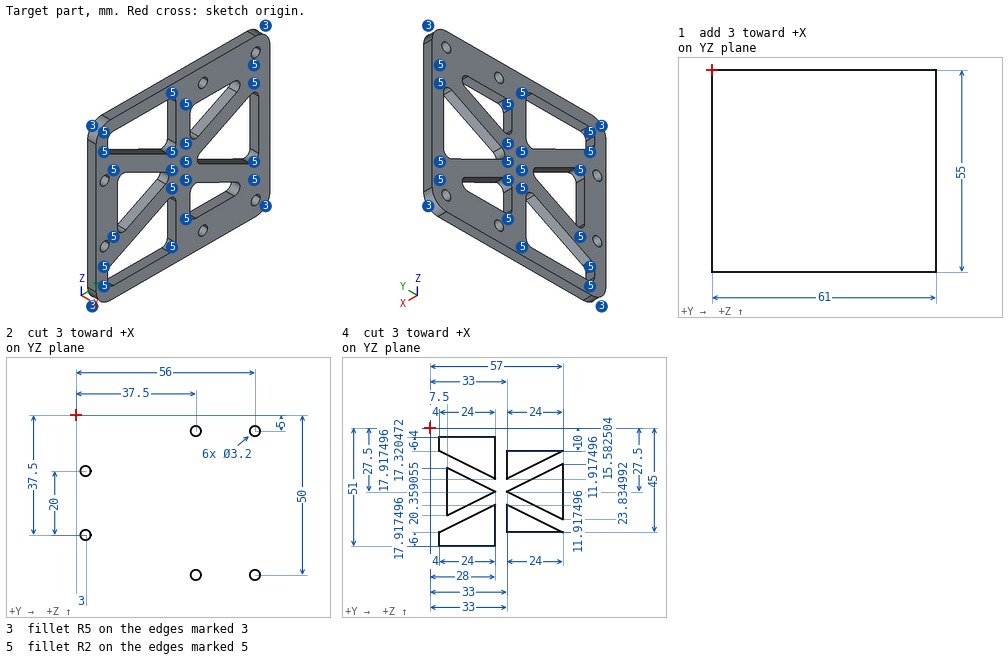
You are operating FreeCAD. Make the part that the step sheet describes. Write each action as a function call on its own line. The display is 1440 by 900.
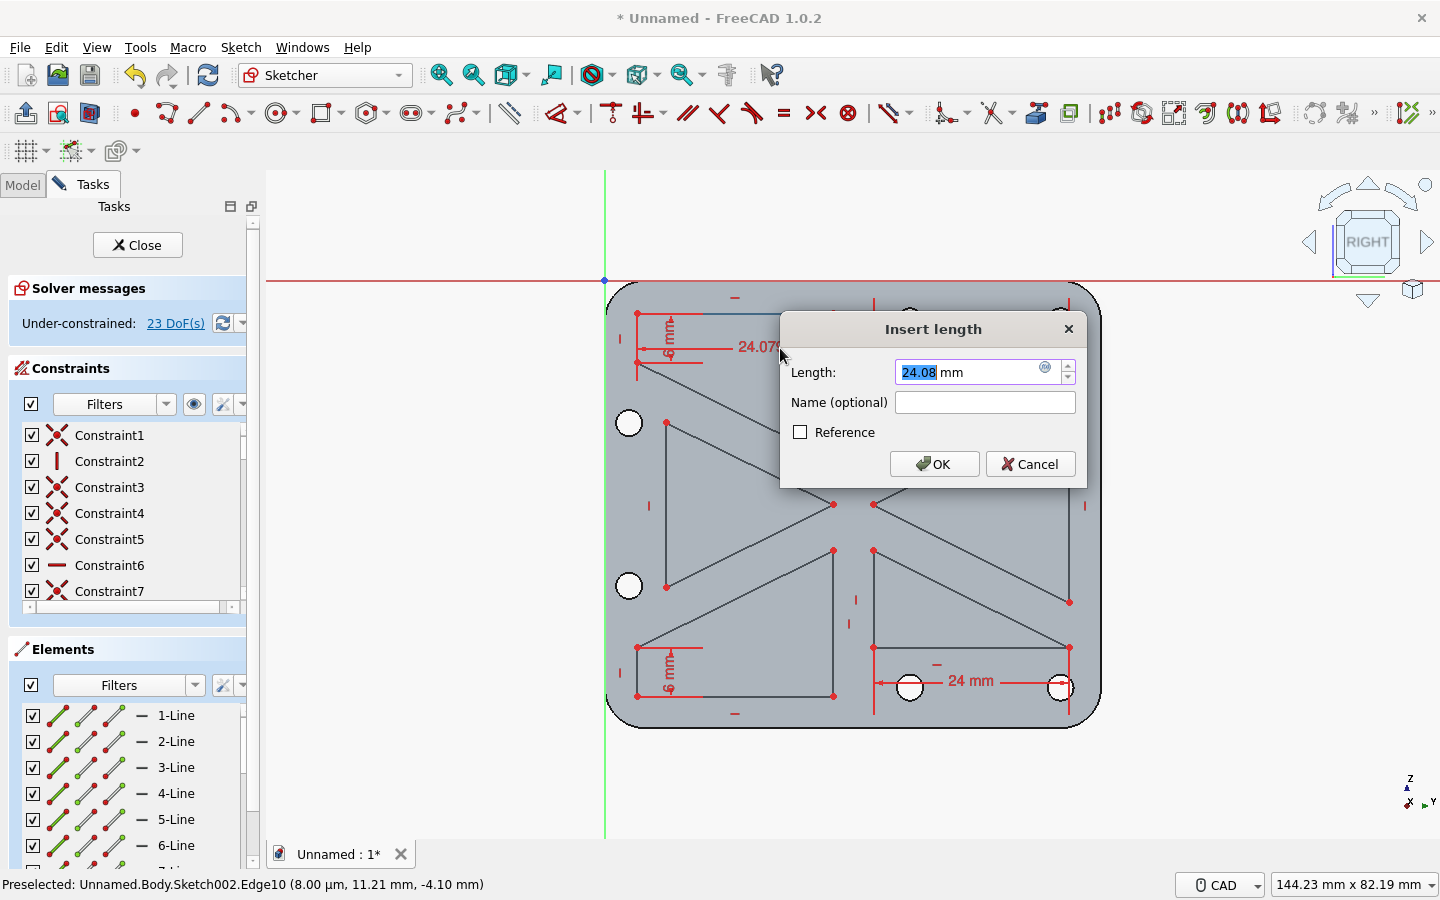
text(24)
key(Return)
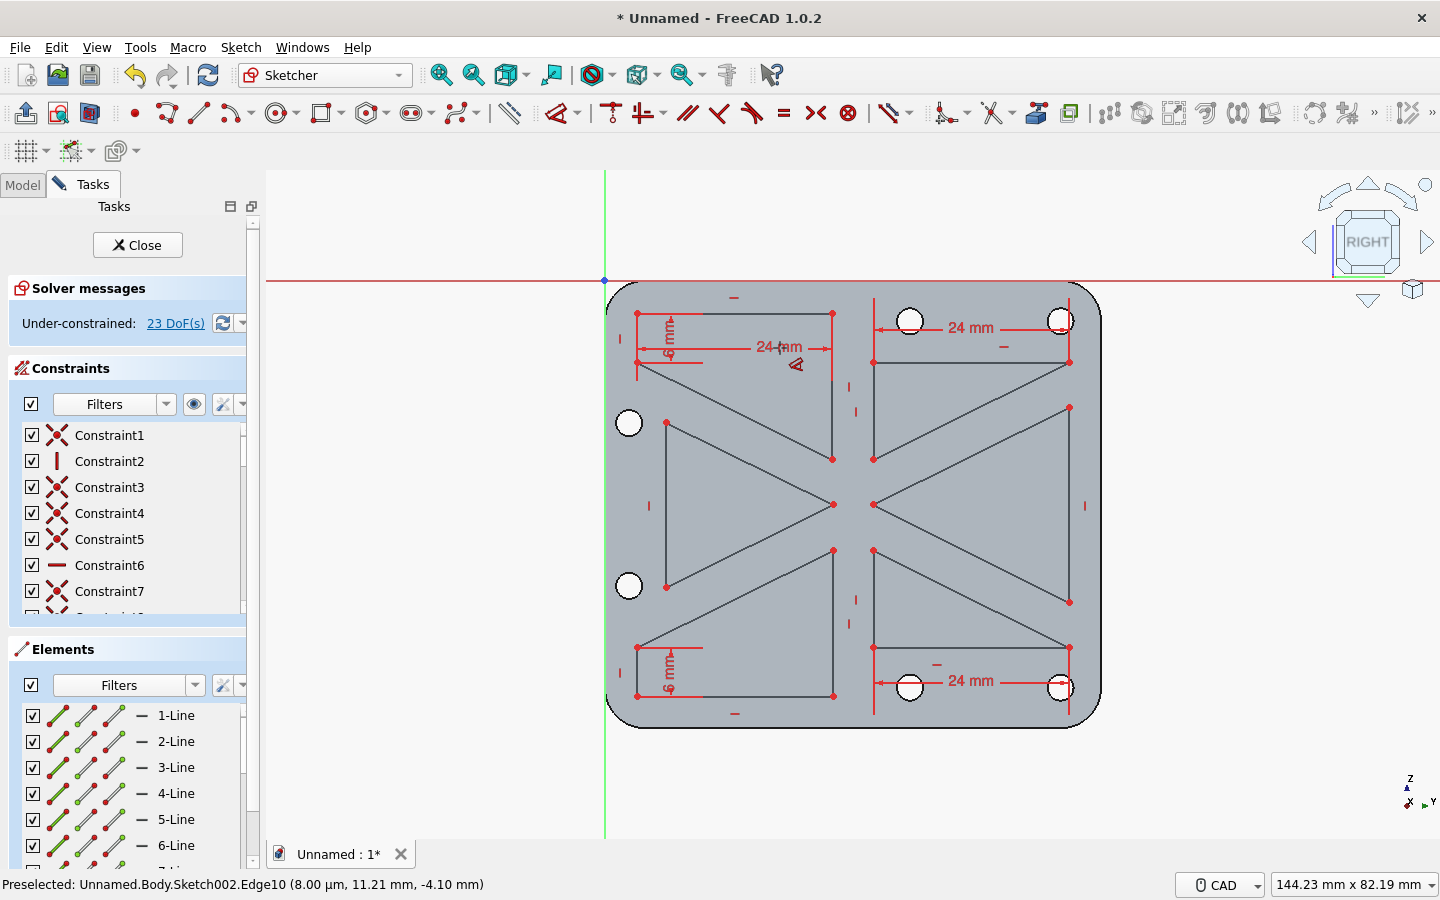
click(774, 697)
click(735, 731)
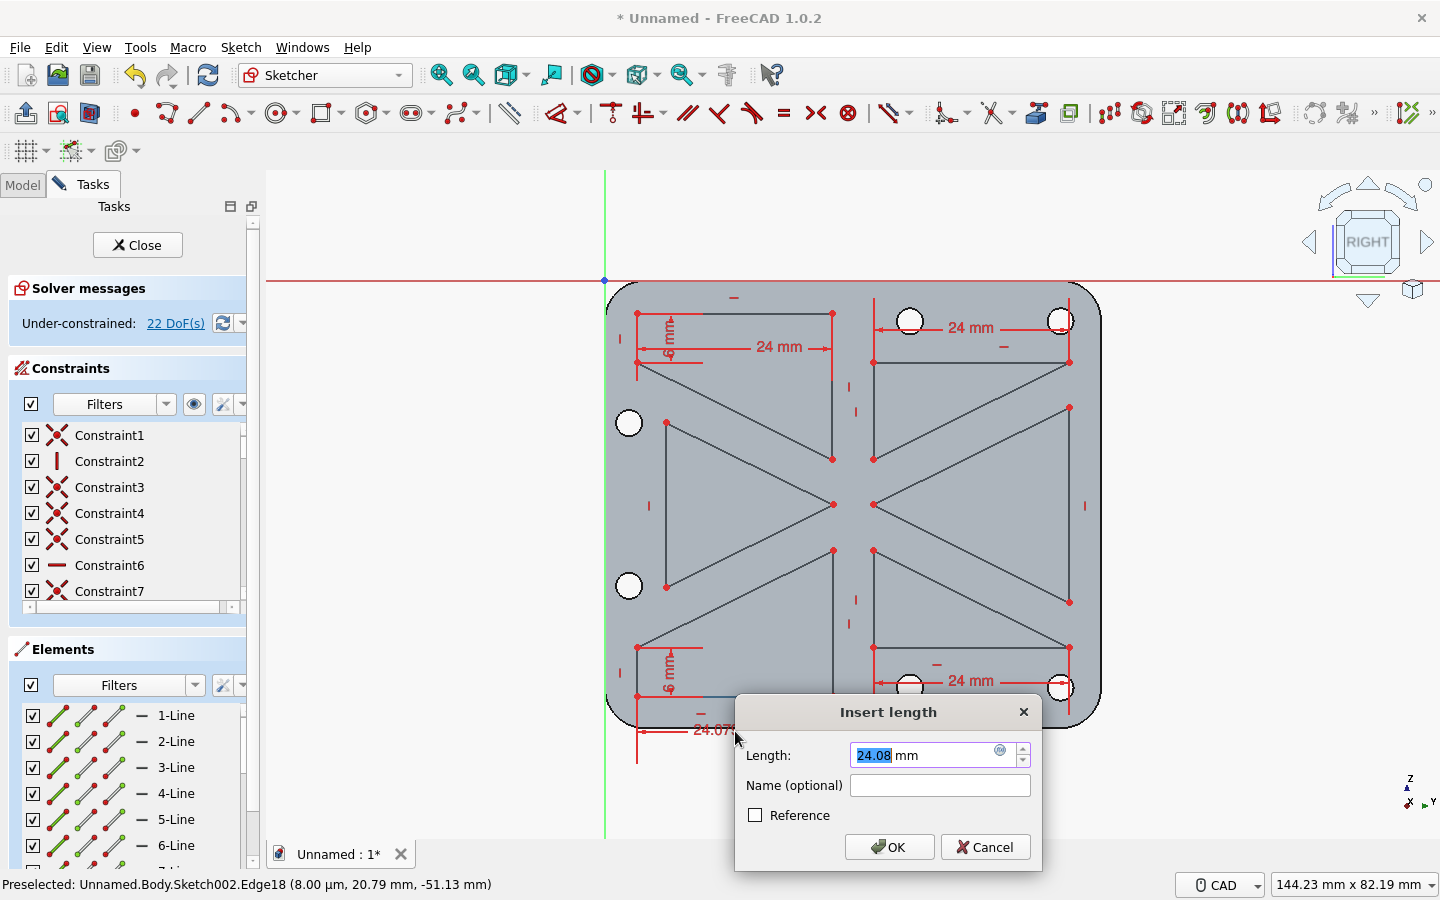
text(24)
key(Return)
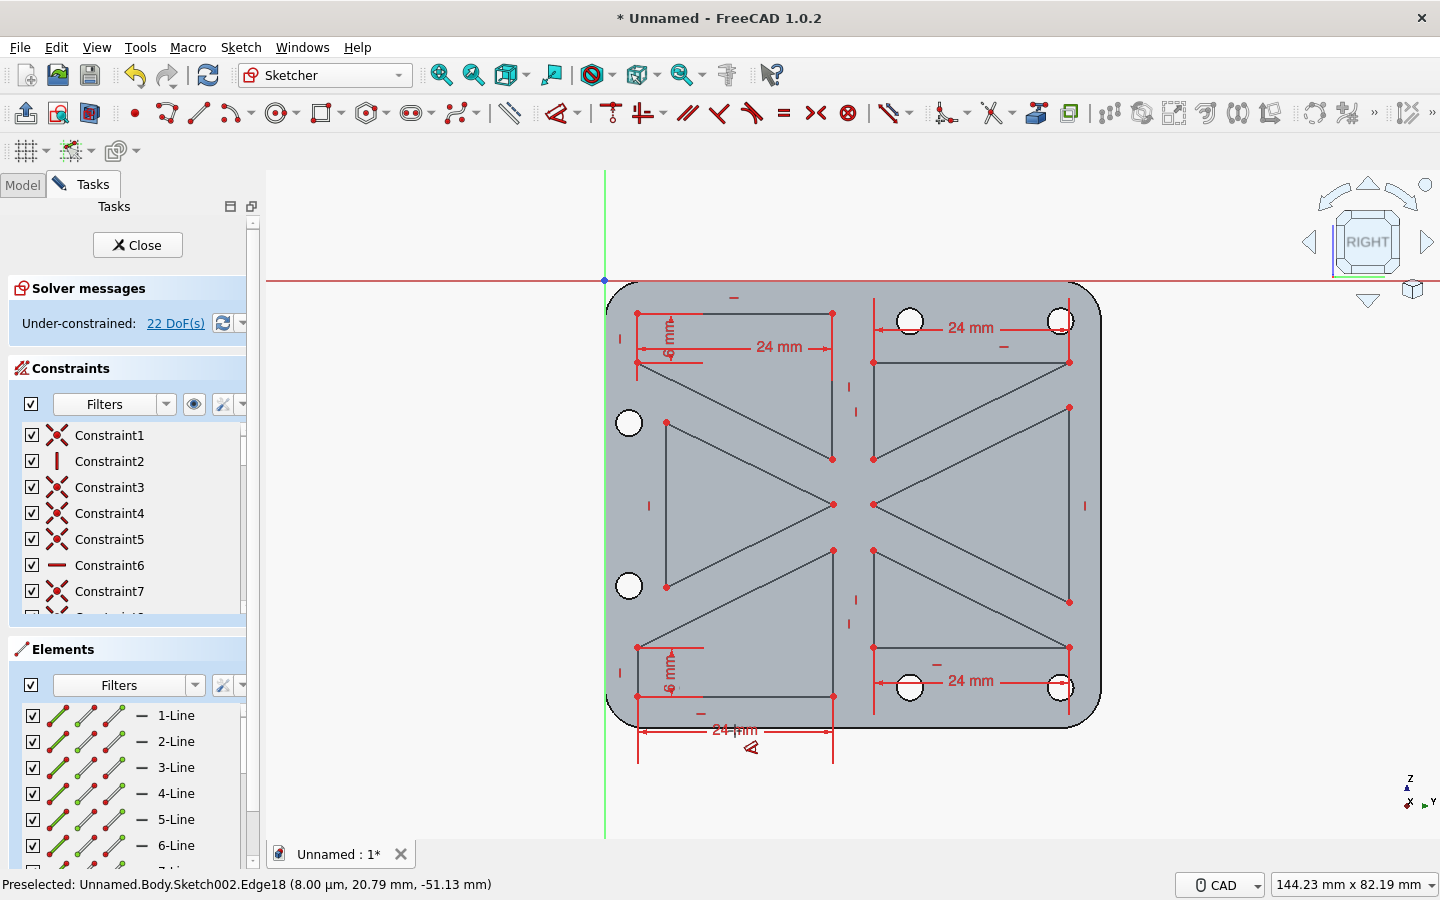
click(637, 314)
click(621, 247)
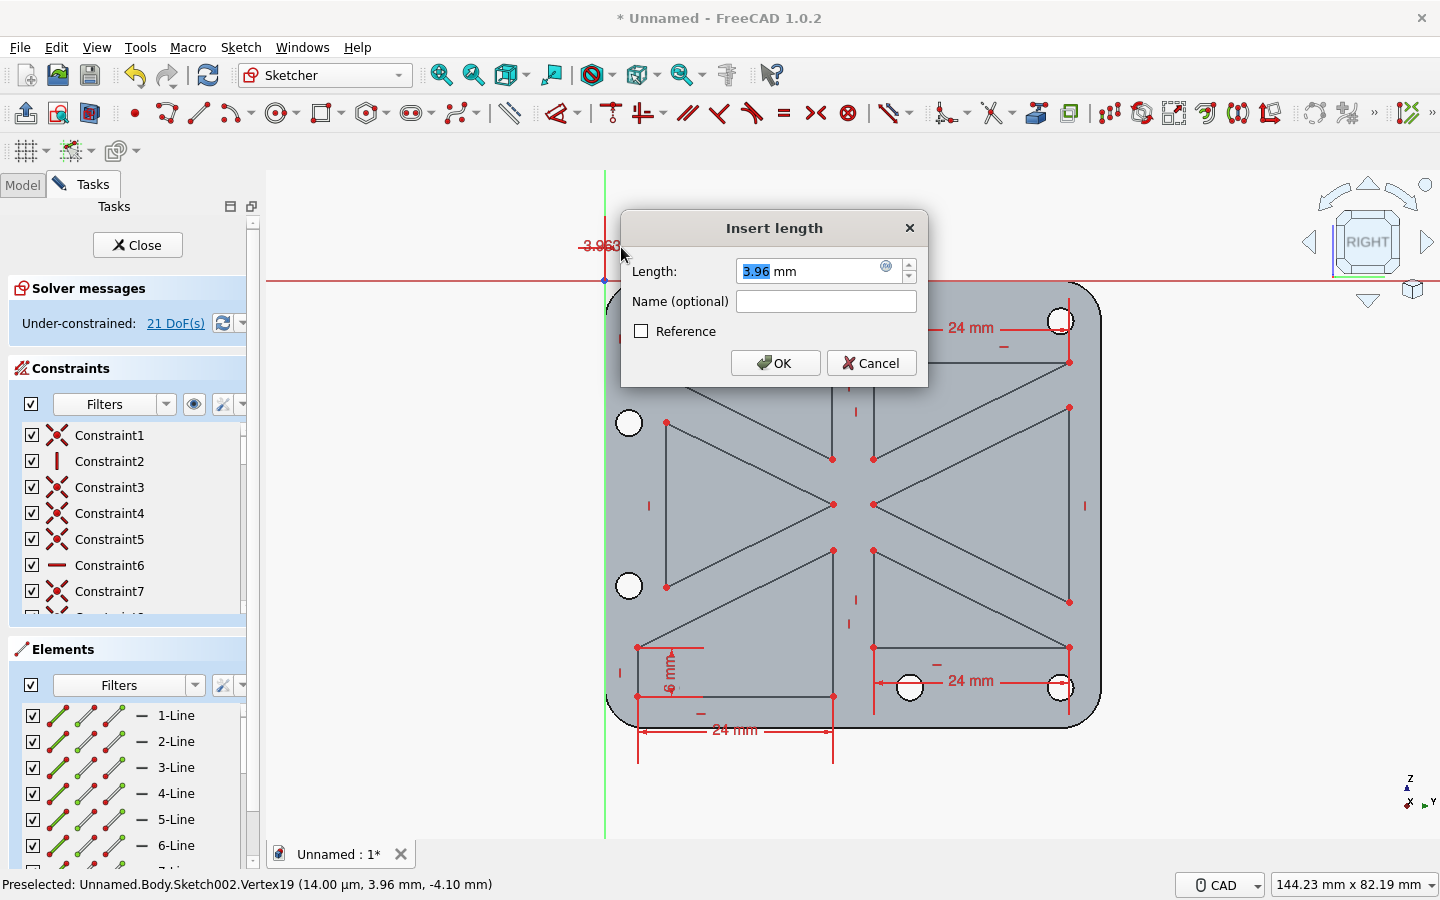
text(4)
key(Return)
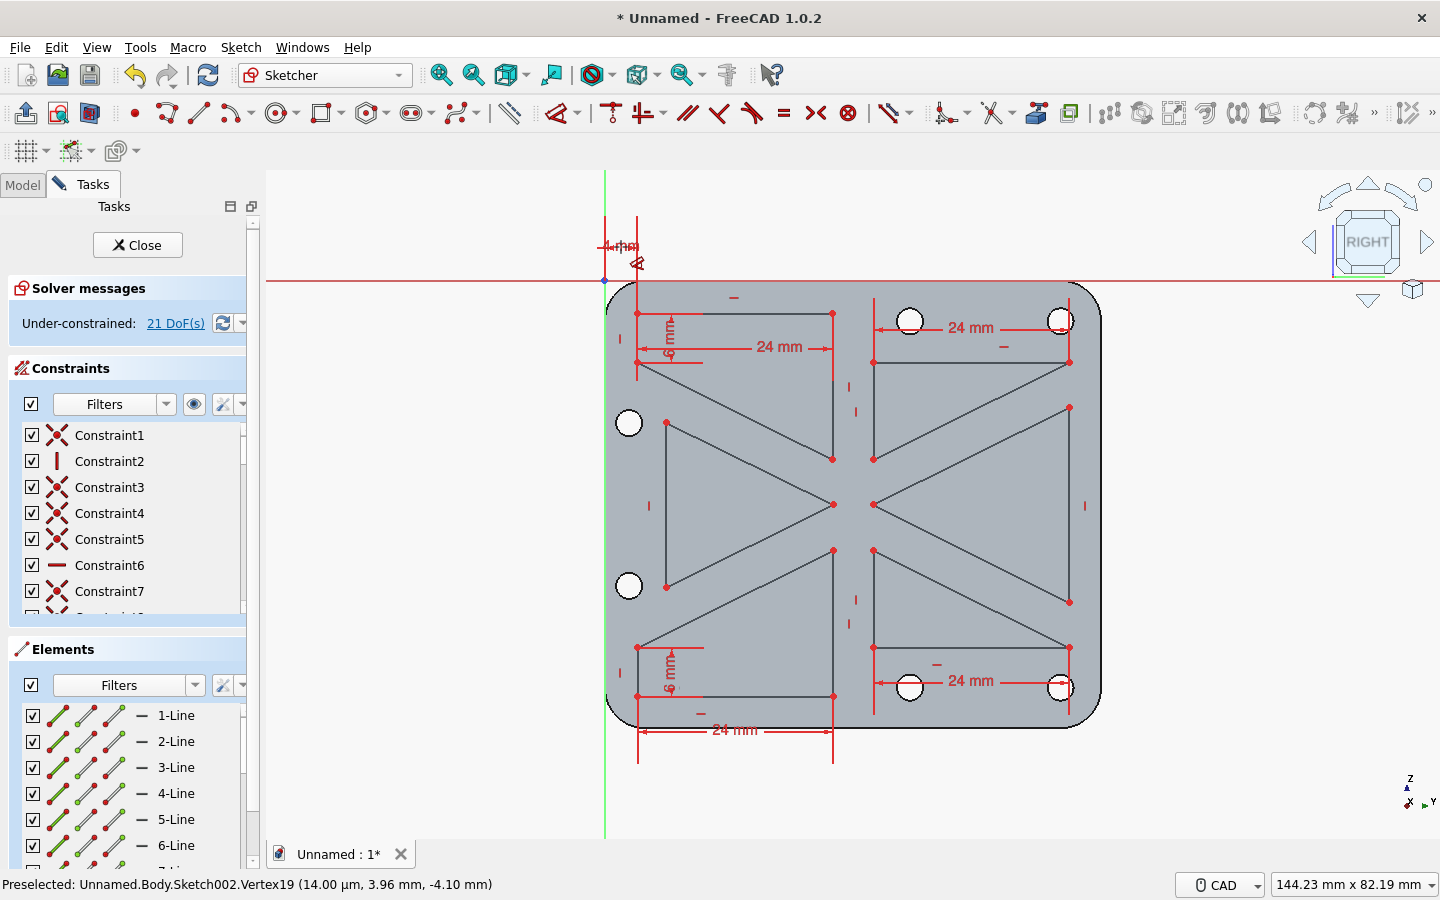
click(637, 314)
click(571, 297)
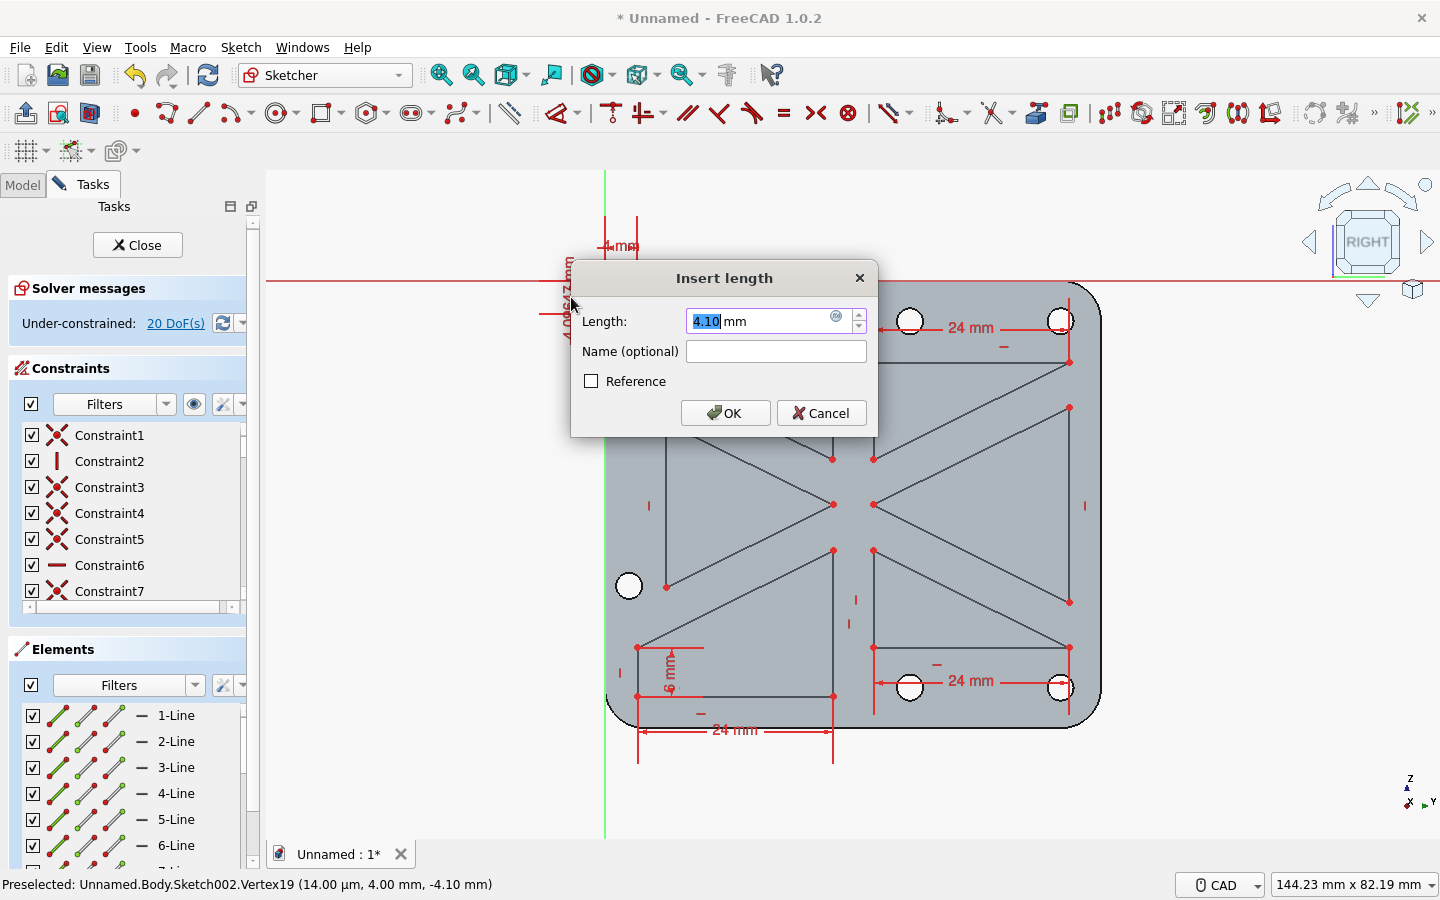
text(4)
key(Return)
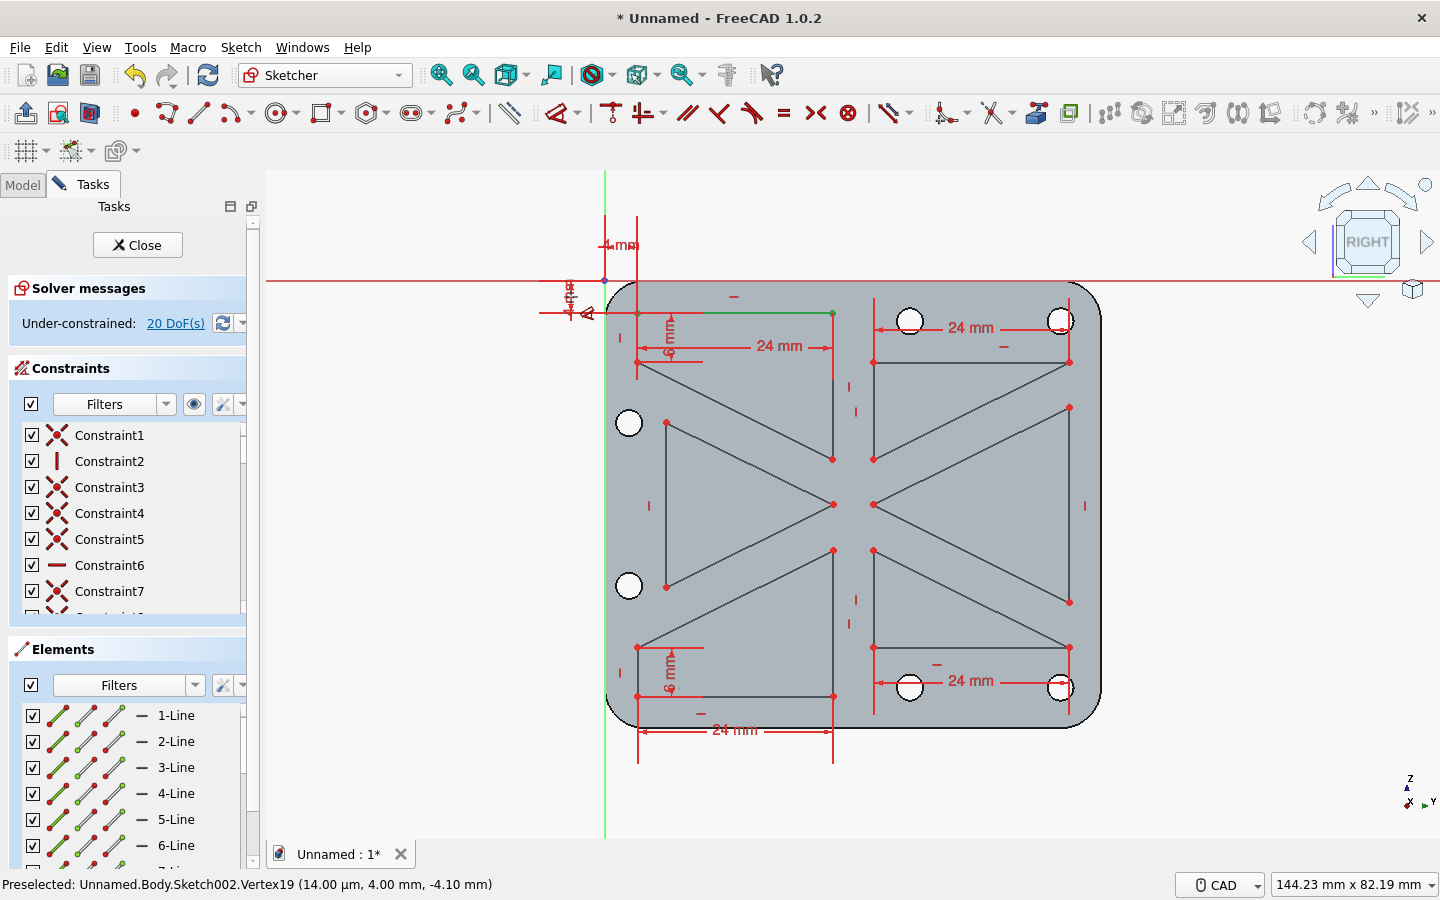
click(638, 697)
click(621, 731)